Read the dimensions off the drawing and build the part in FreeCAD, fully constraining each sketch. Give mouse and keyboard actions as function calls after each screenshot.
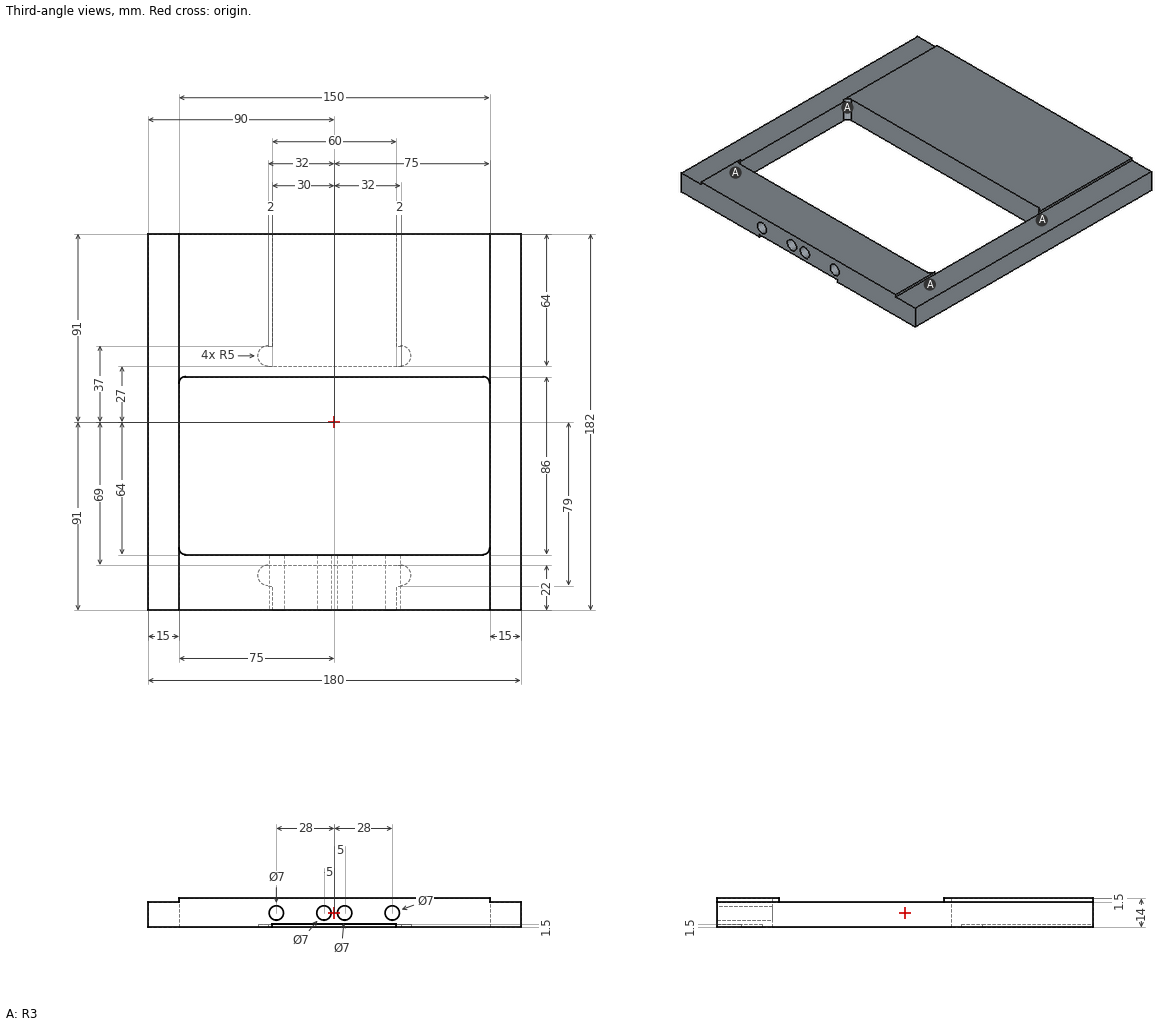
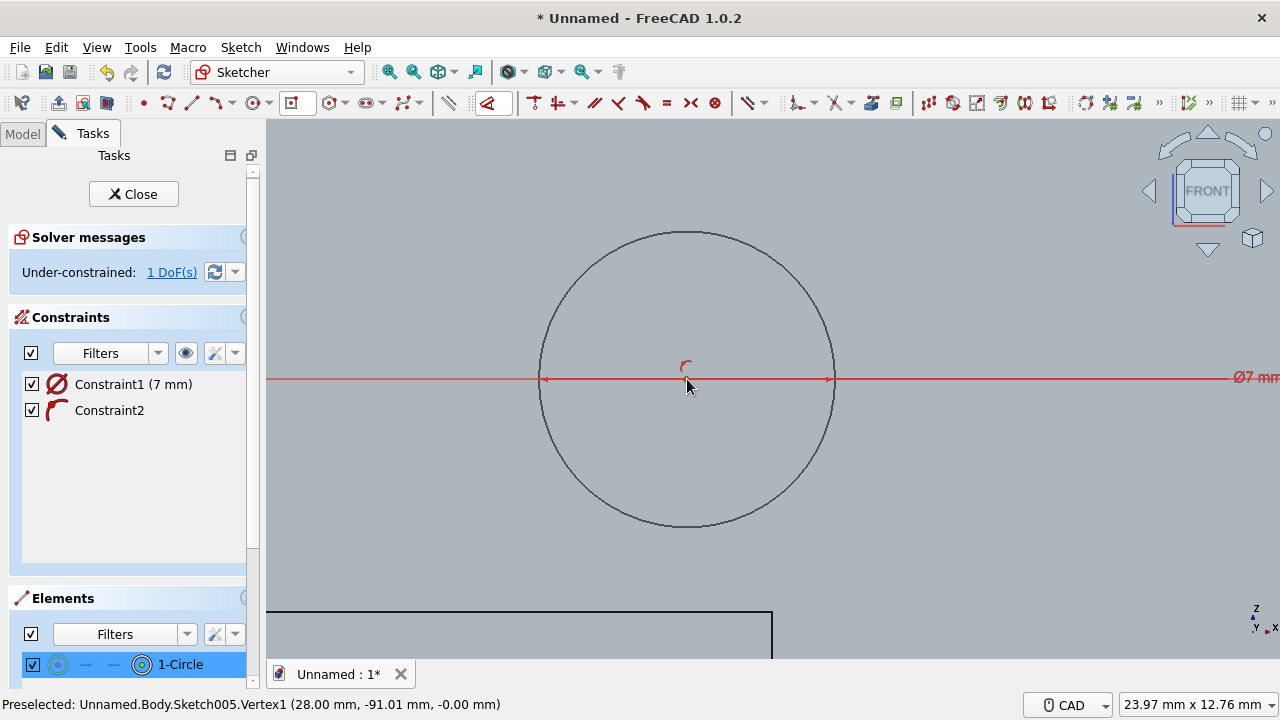
key(l)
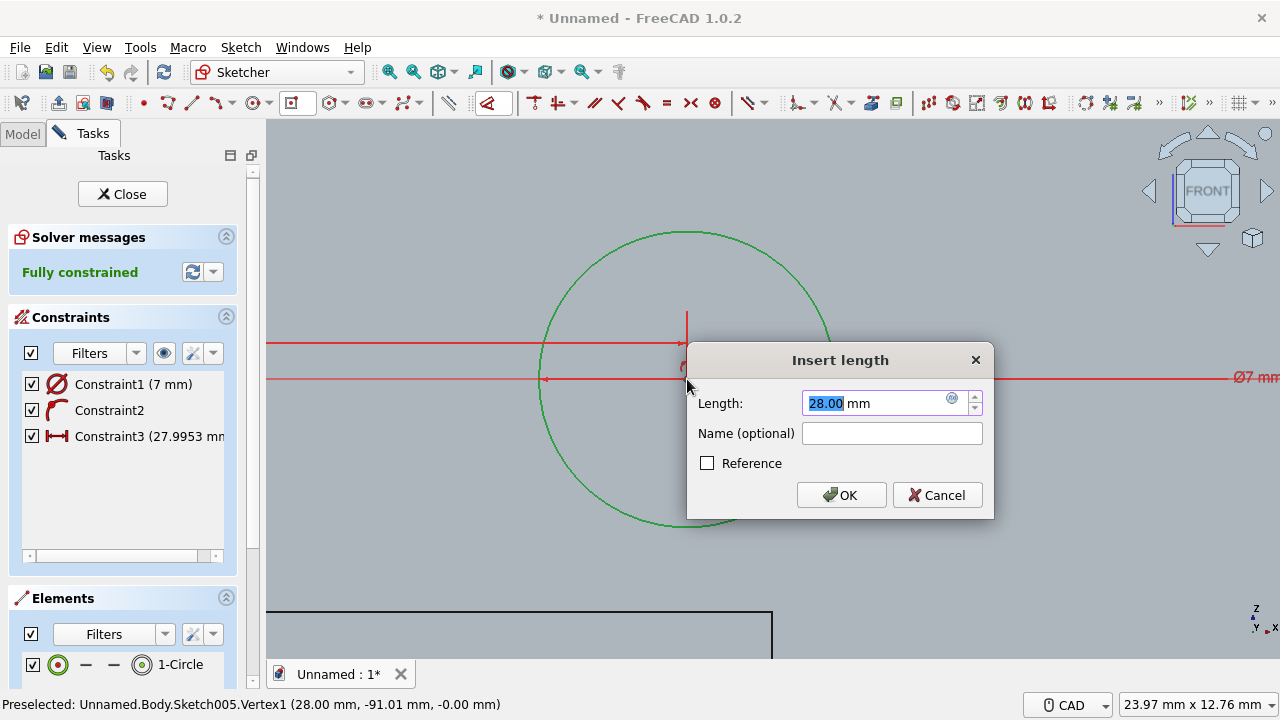
text(28)
key(Return)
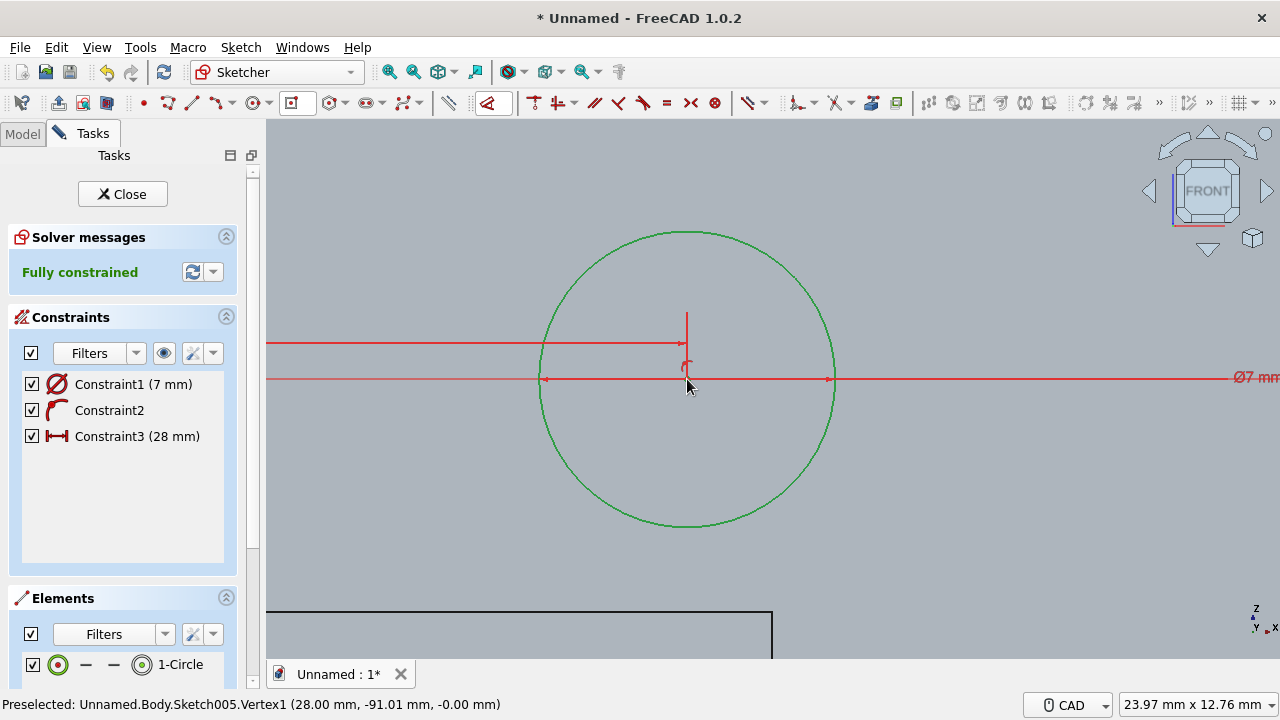
click(123, 194)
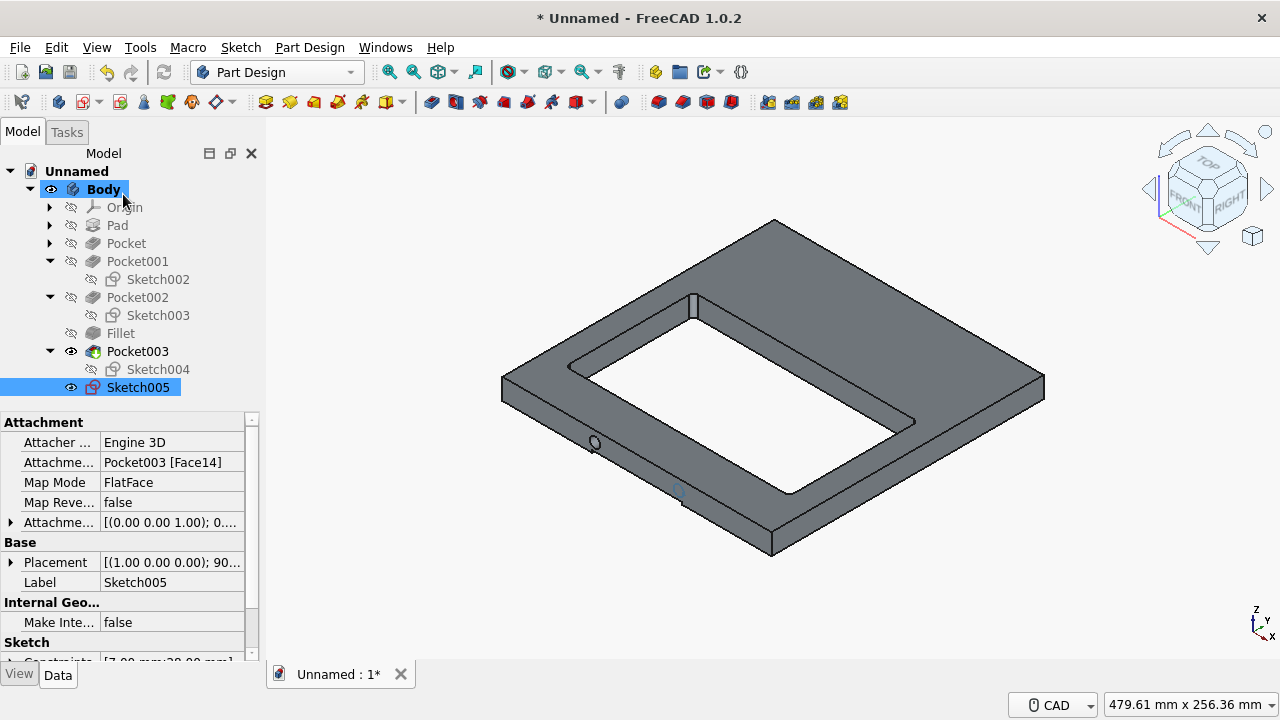
click(432, 102)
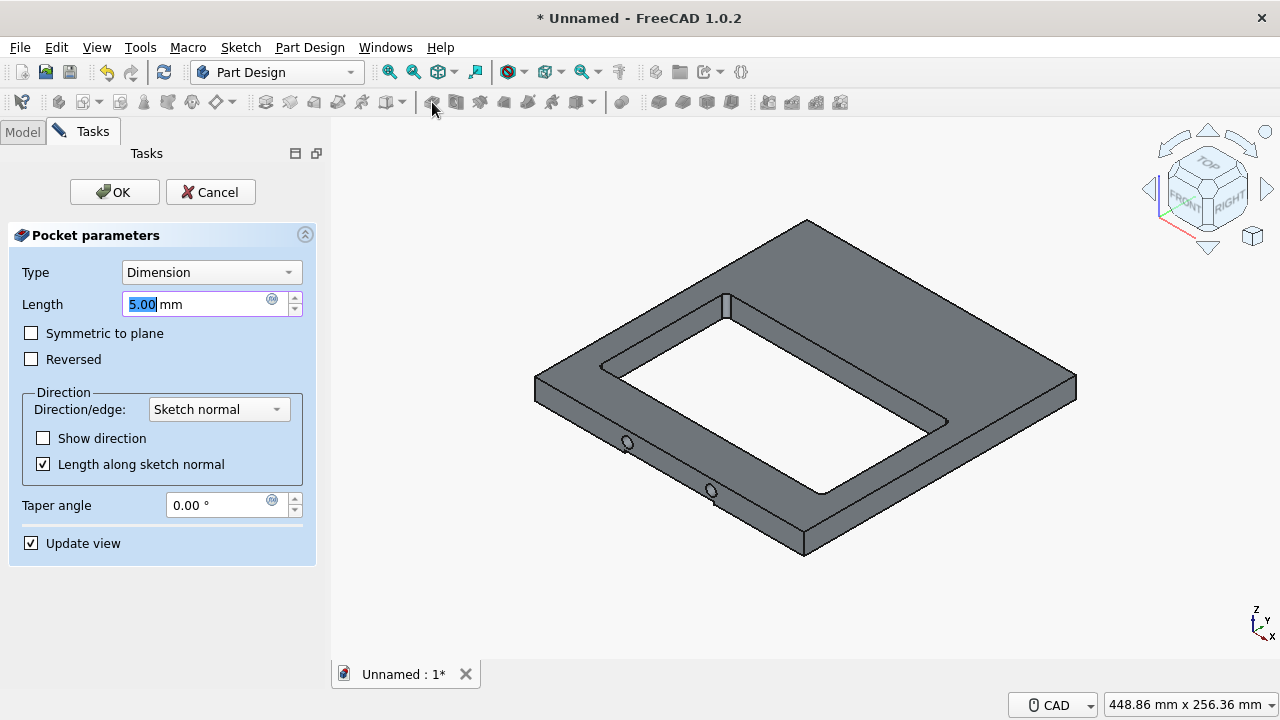
click(212, 272)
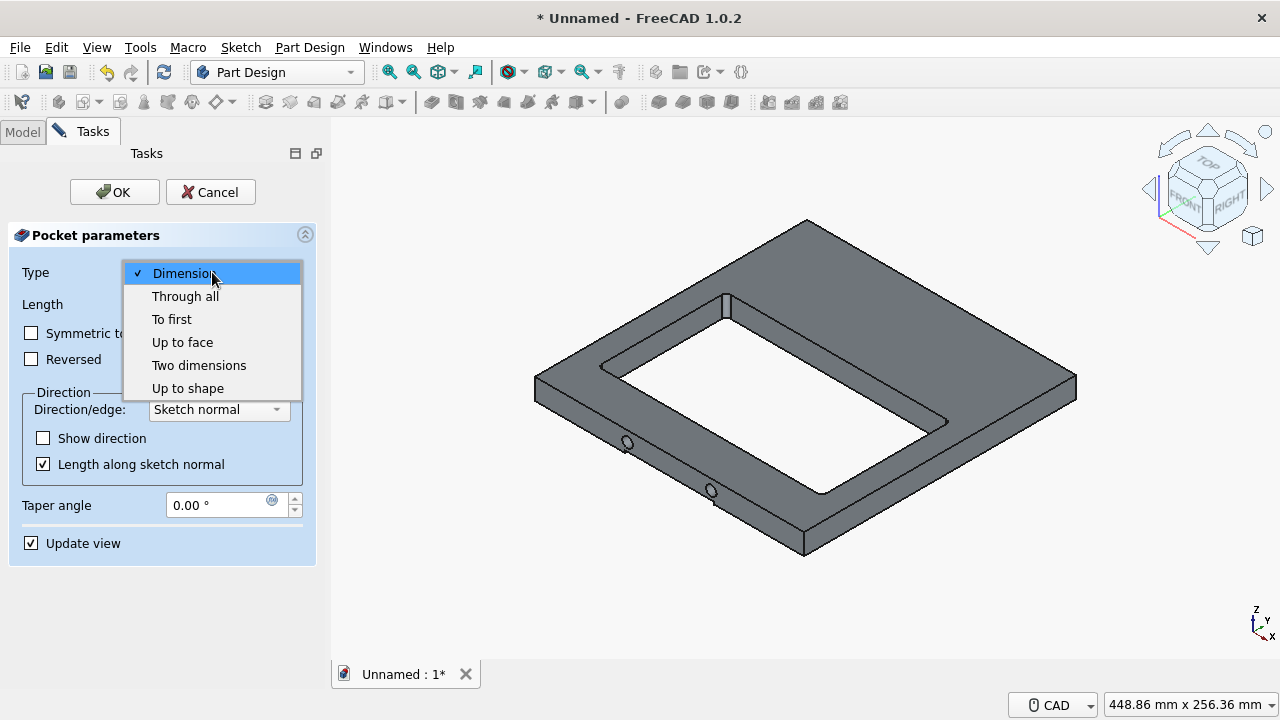
click(212, 320)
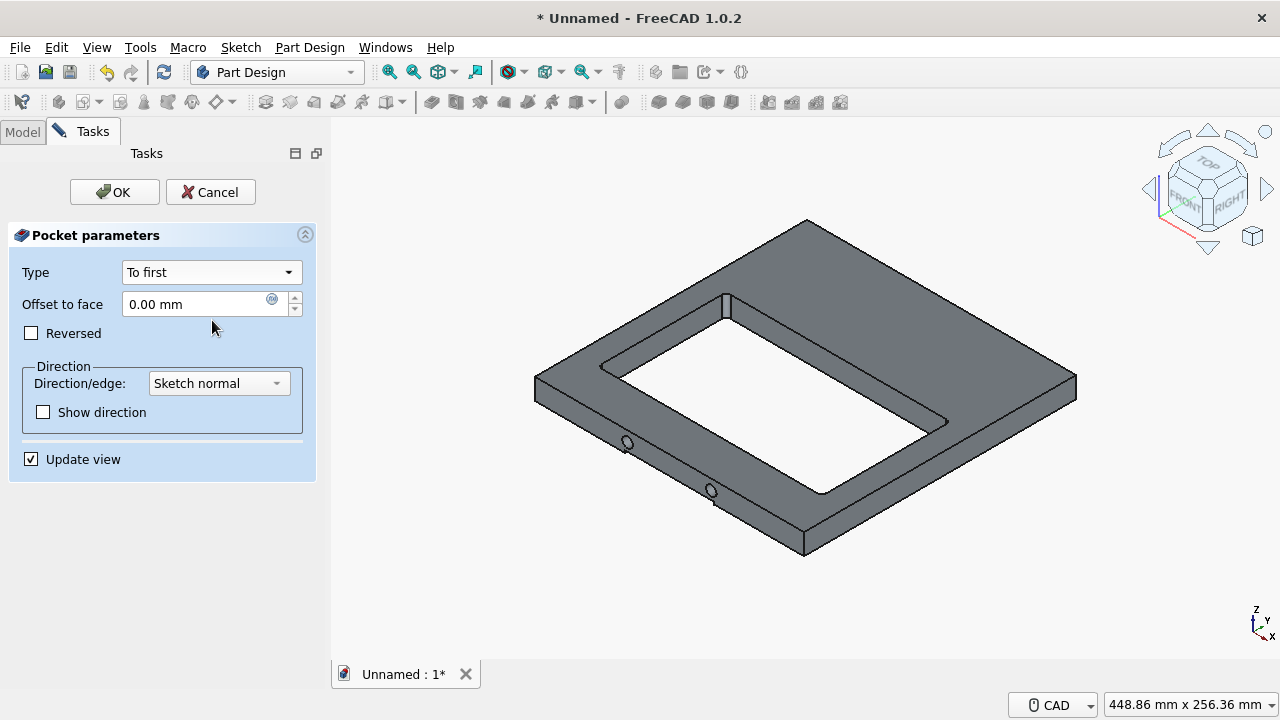
click(115, 192)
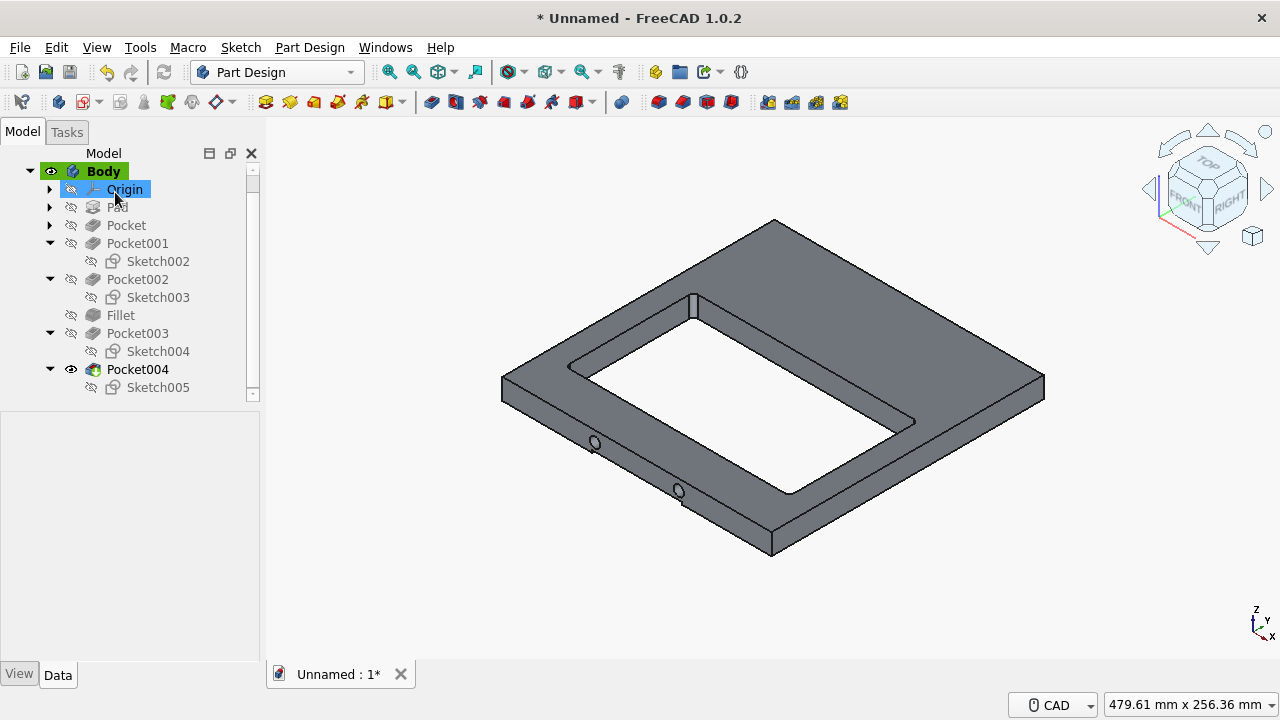
click(752, 532)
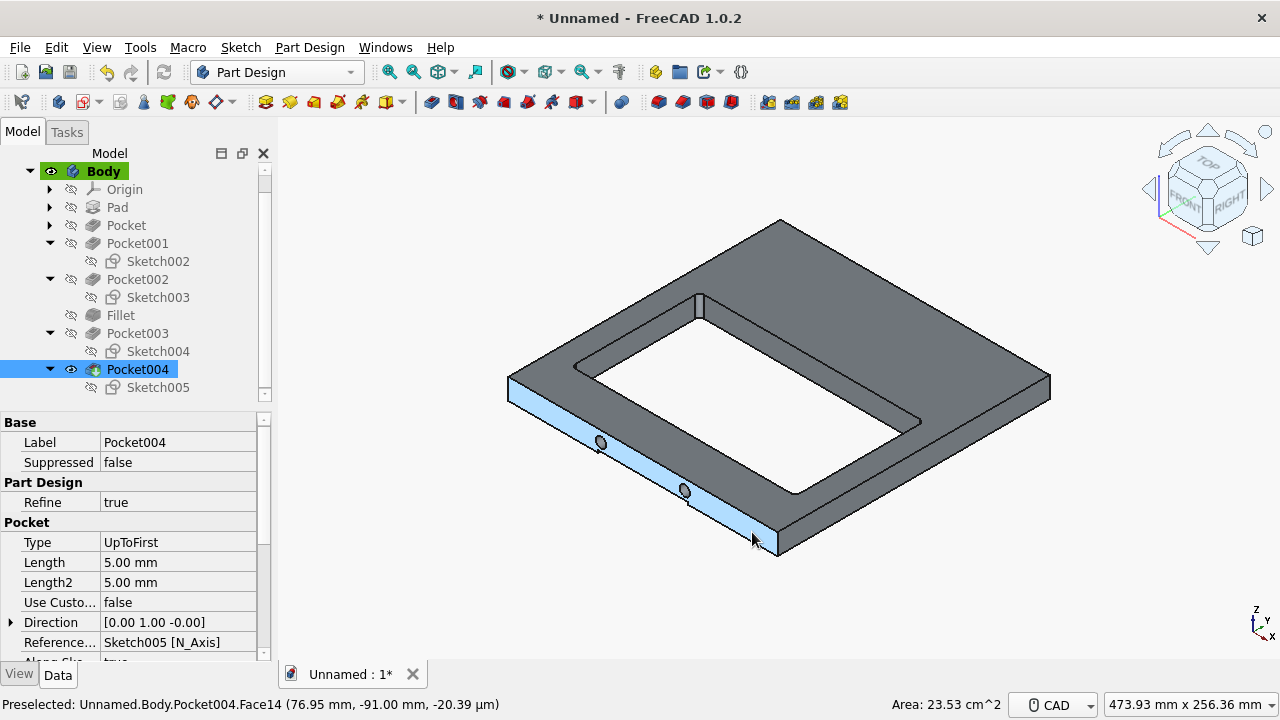
click(84, 102)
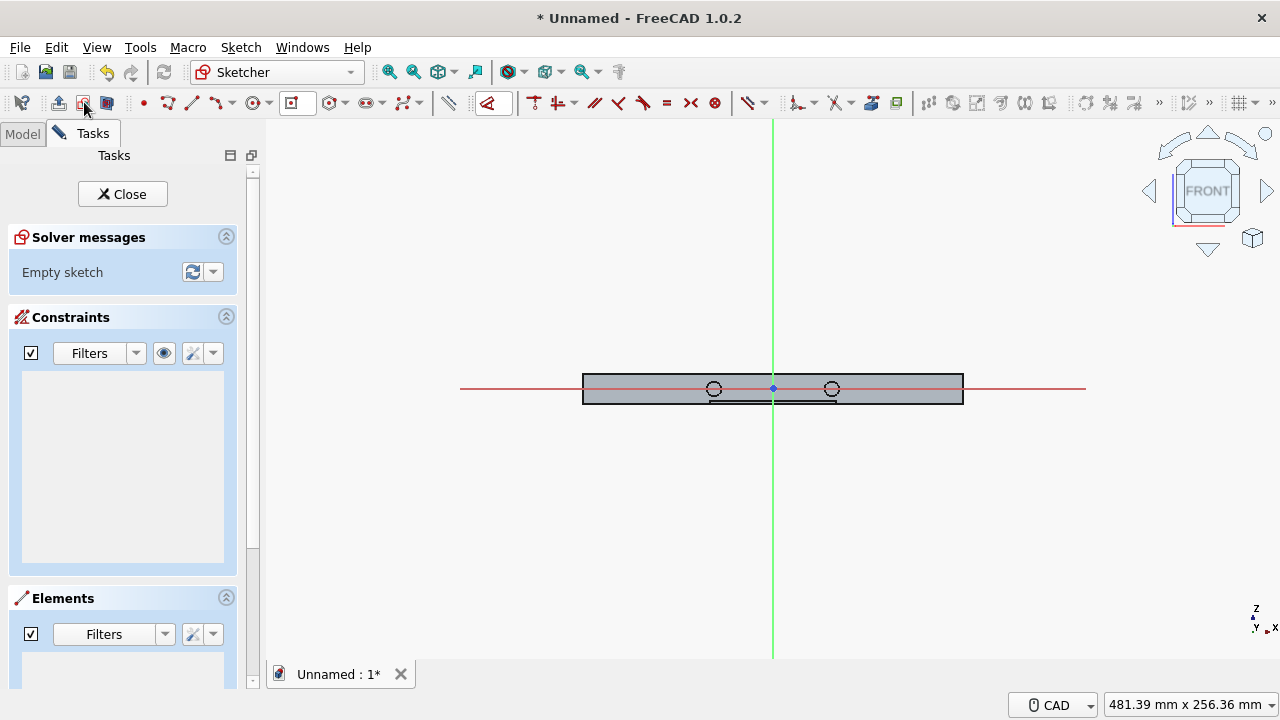
scroll(767, 389, up, 15)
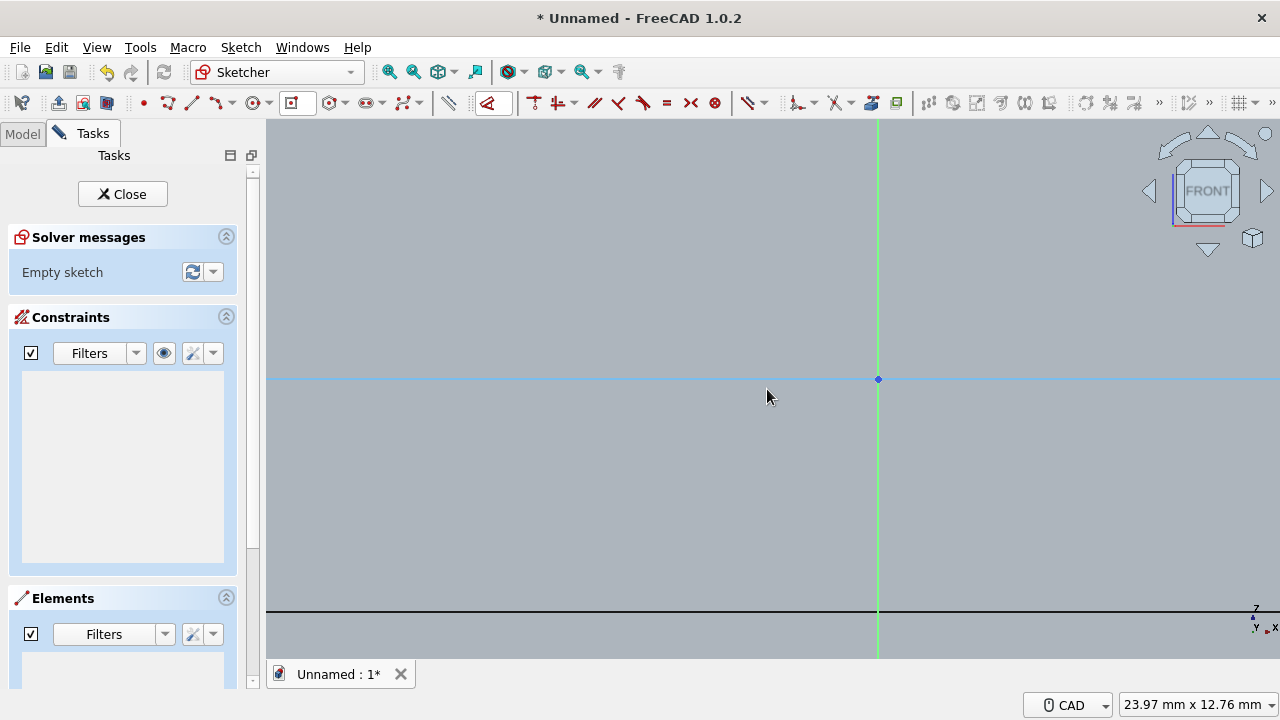
key(g)
key(c)